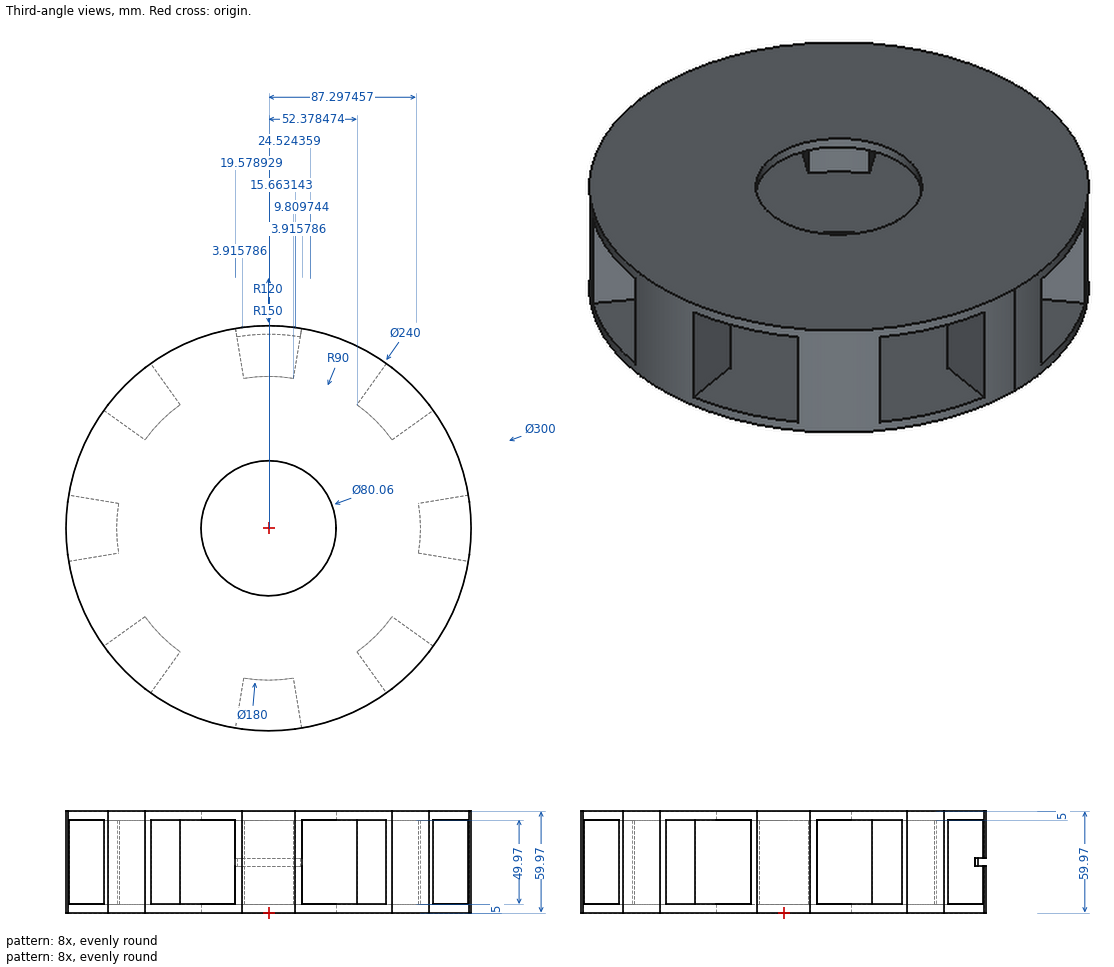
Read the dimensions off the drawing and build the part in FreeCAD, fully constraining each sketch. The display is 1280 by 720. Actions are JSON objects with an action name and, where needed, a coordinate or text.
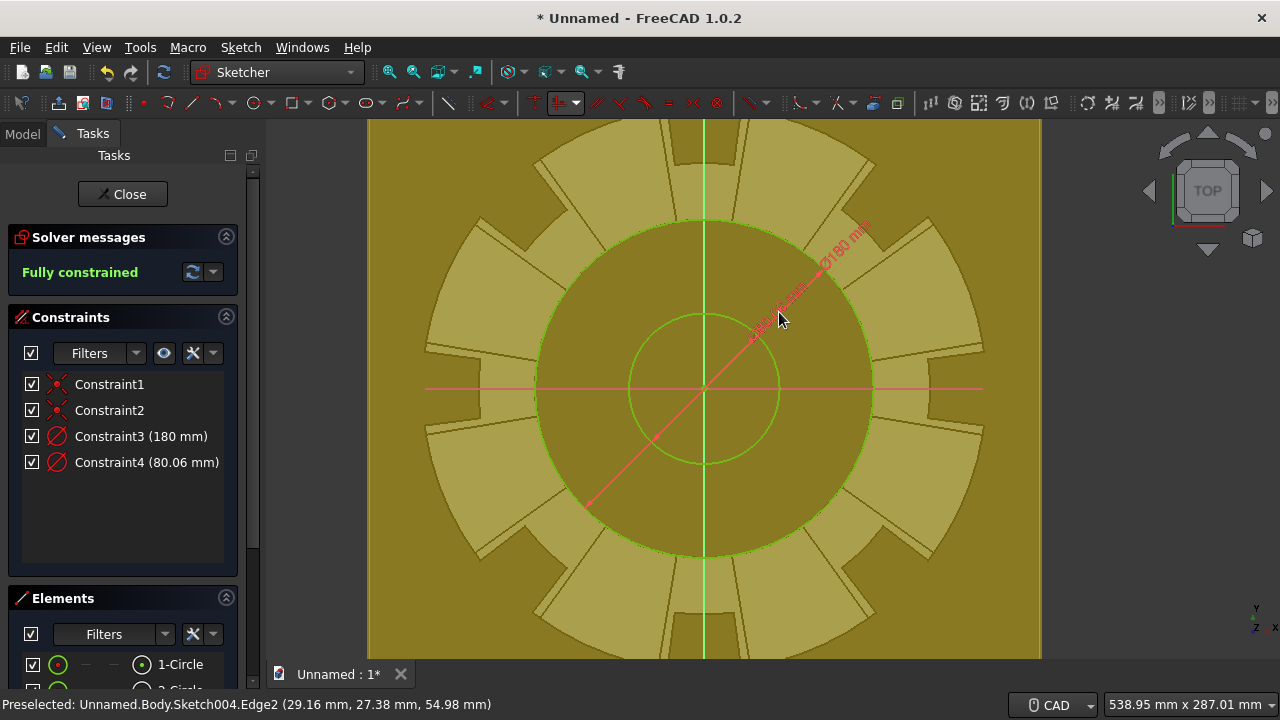
{"action": "left_click", "coordinate": [123, 194]}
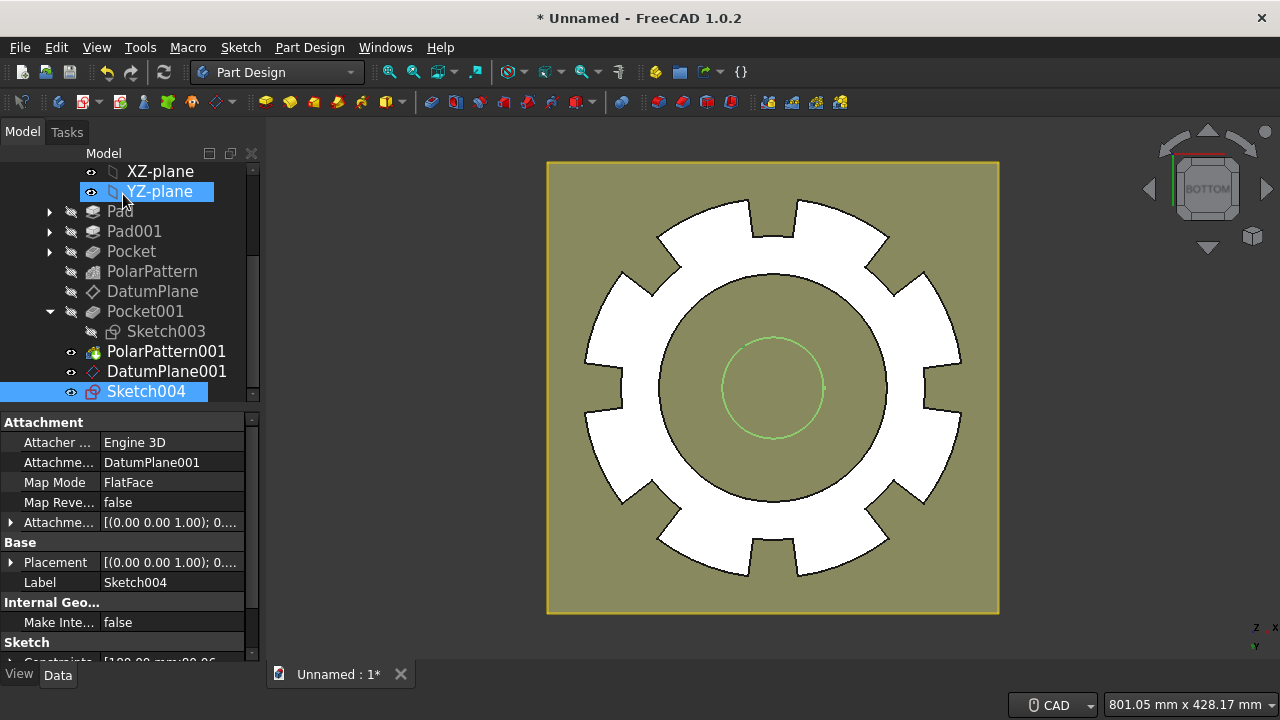
{"action": "left_click", "coordinate": [266, 102]}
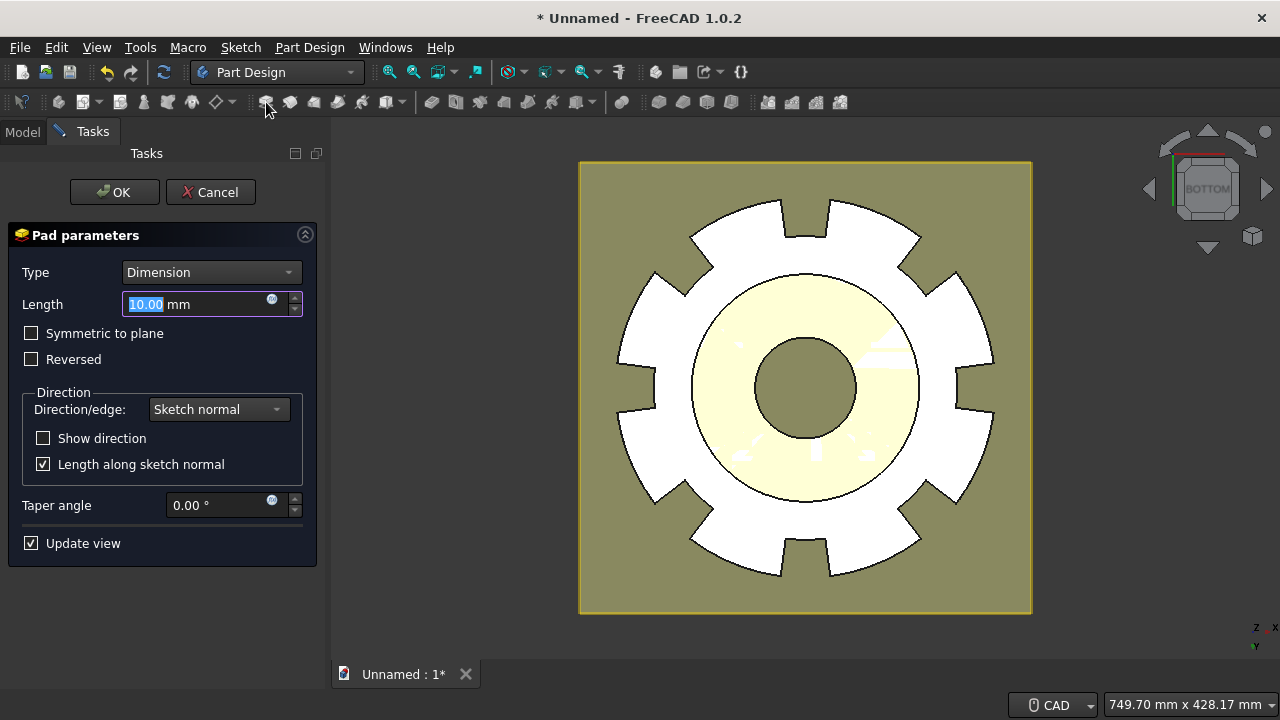
{"action": "type", "text": "5"}
{"action": "key", "text": "Tab"}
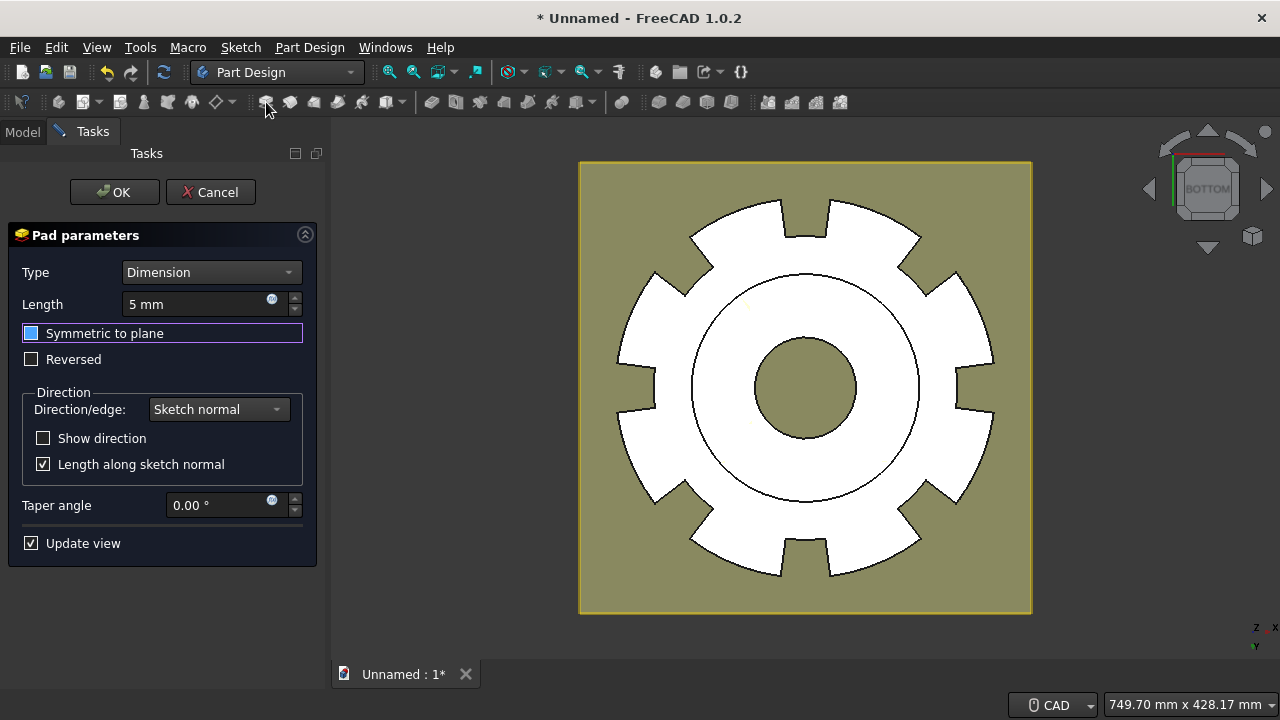
{"action": "left_click", "coordinate": [115, 192]}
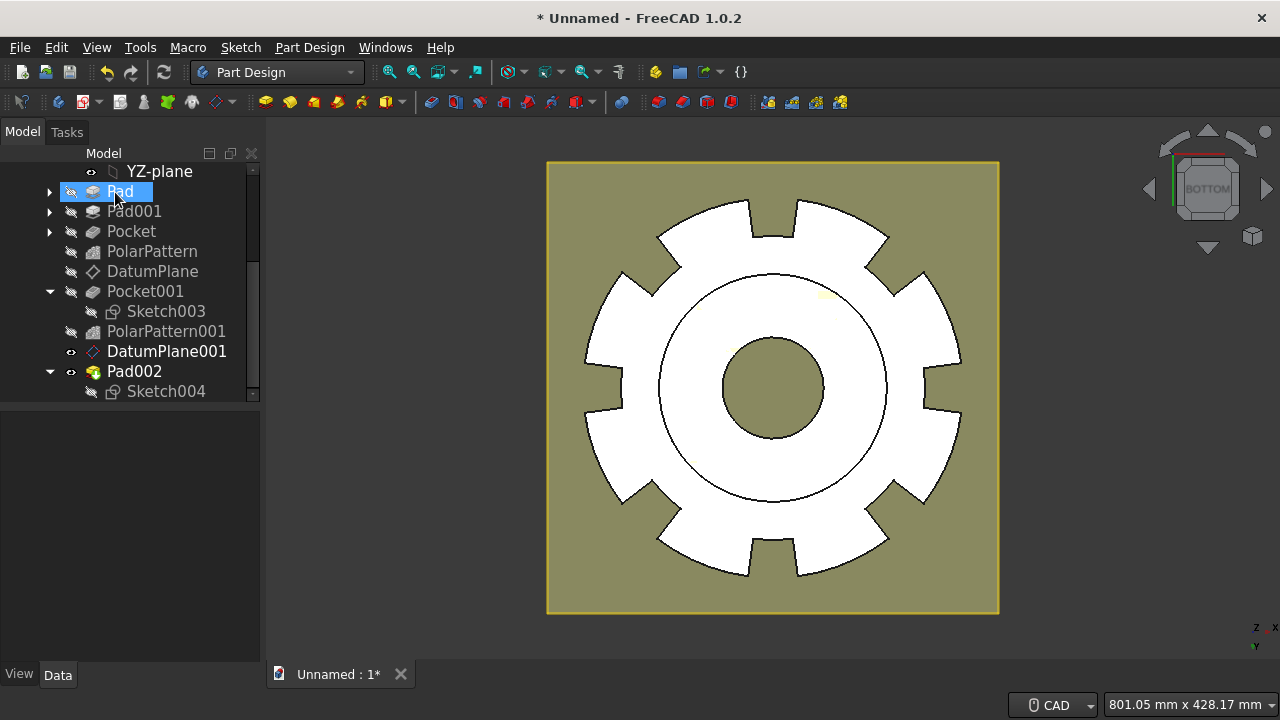
{"action": "left_click", "coordinate": [116, 352]}
{"action": "key", "text": "space"}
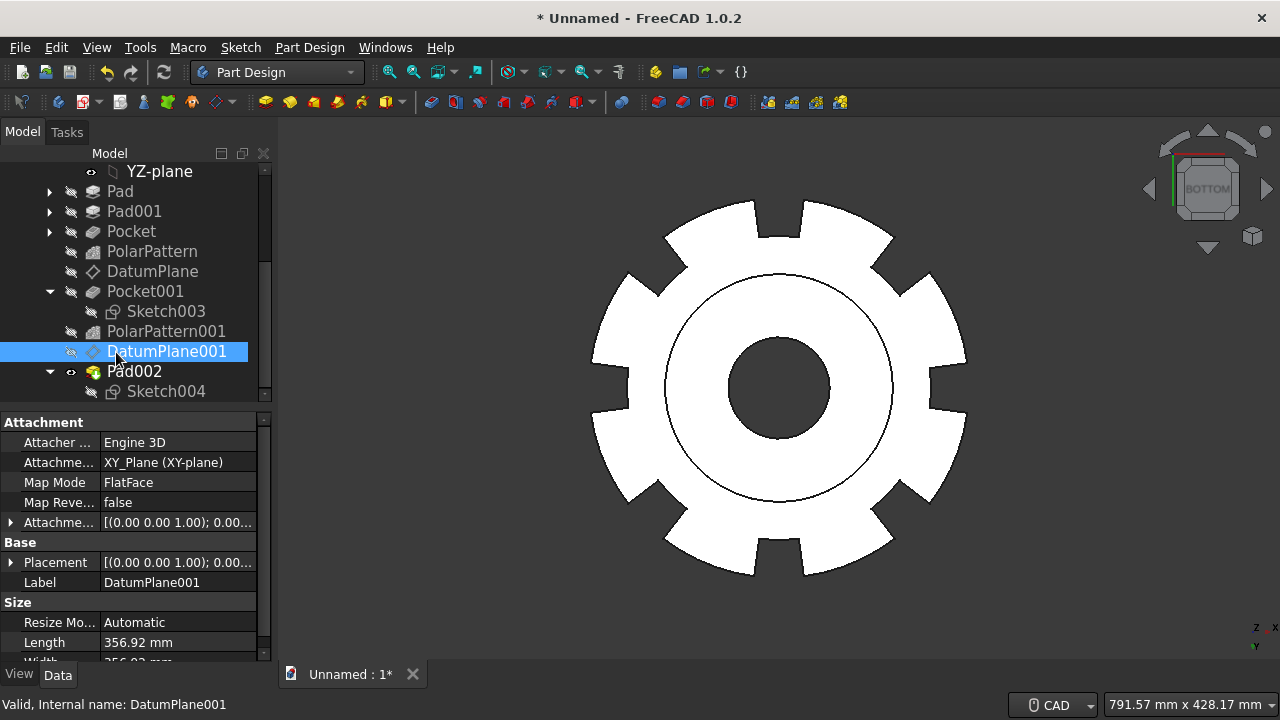
{"action": "left_click", "coordinate": [318, 619]}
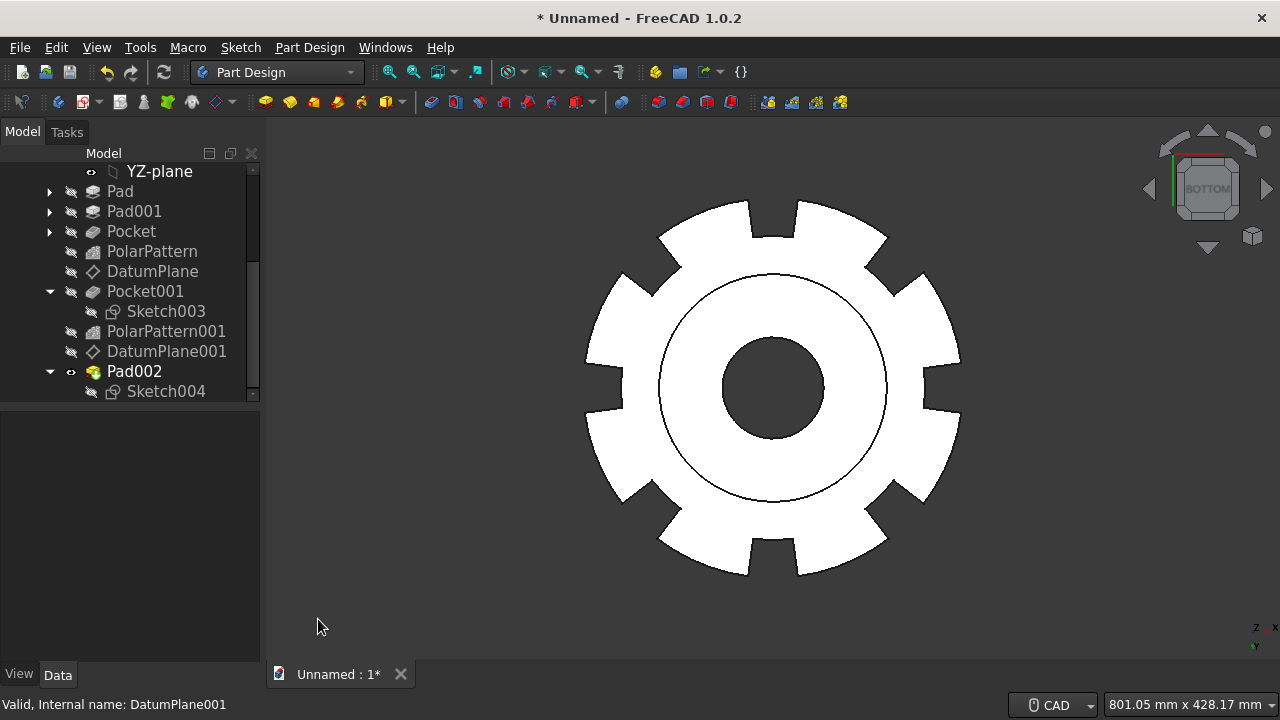
{"action": "left_click", "coordinate": [84, 102]}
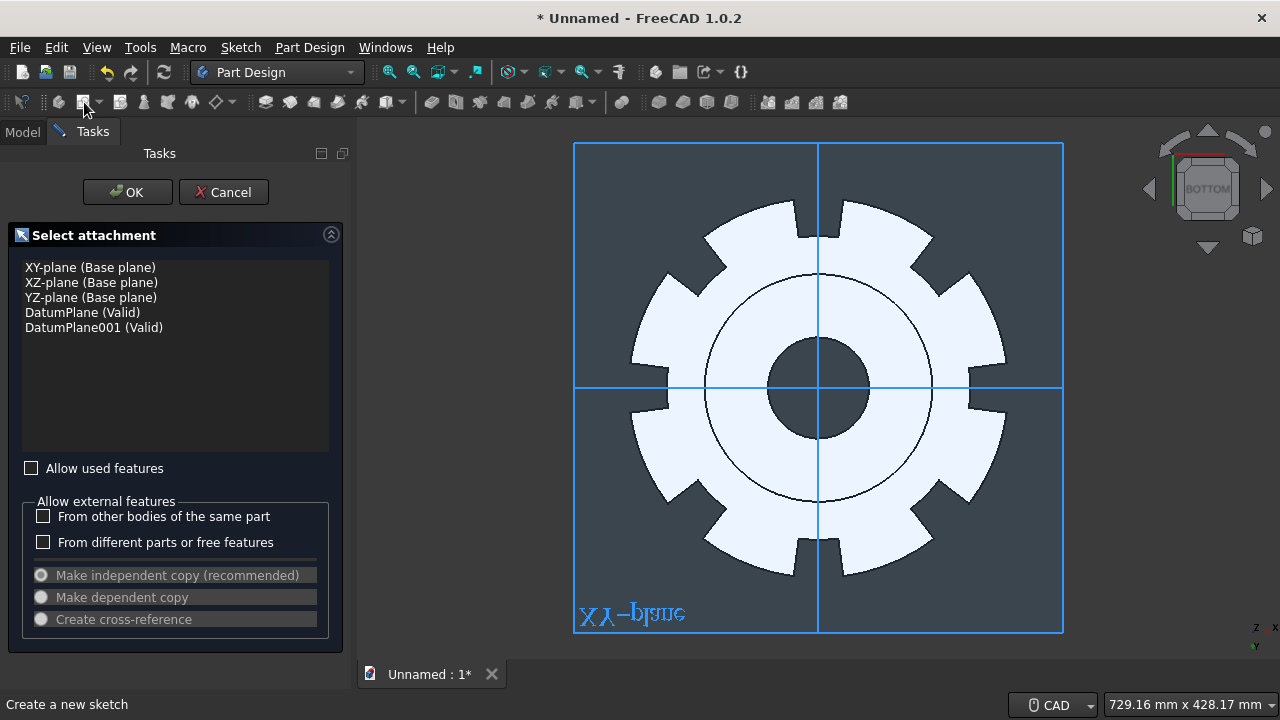
{"action": "left_click", "coordinate": [82, 268]}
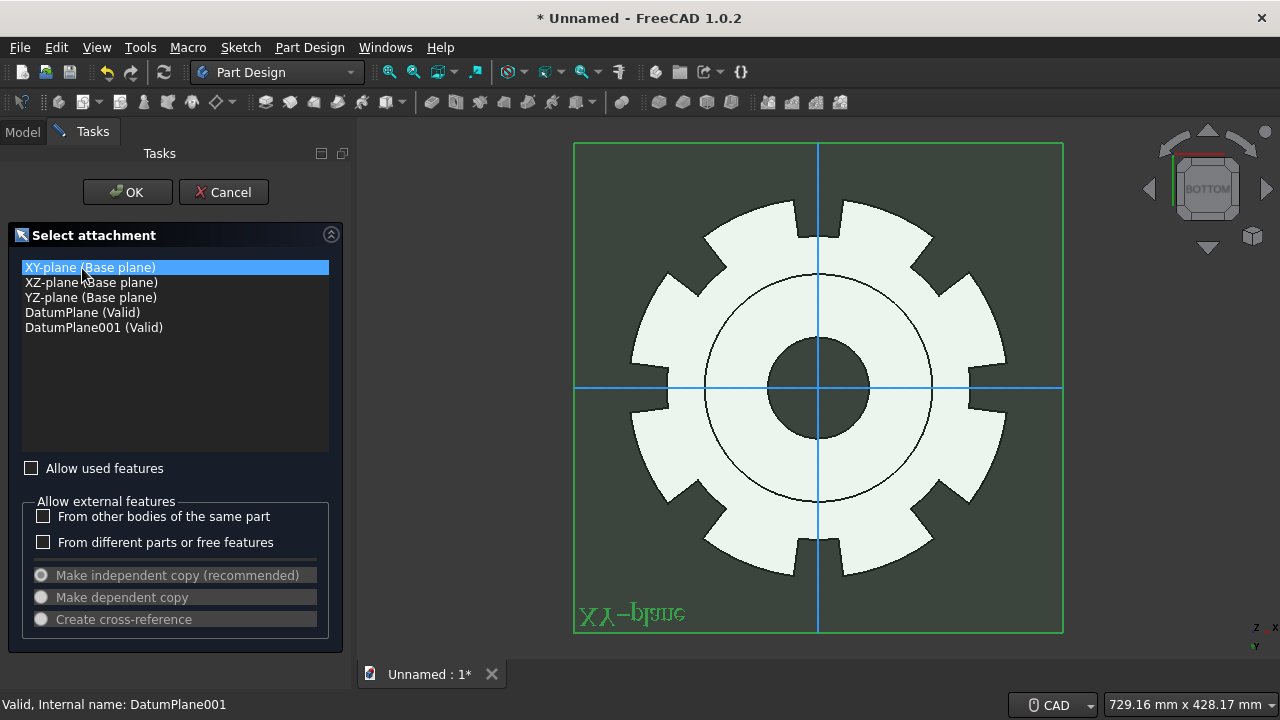
{"action": "left_click", "coordinate": [128, 192]}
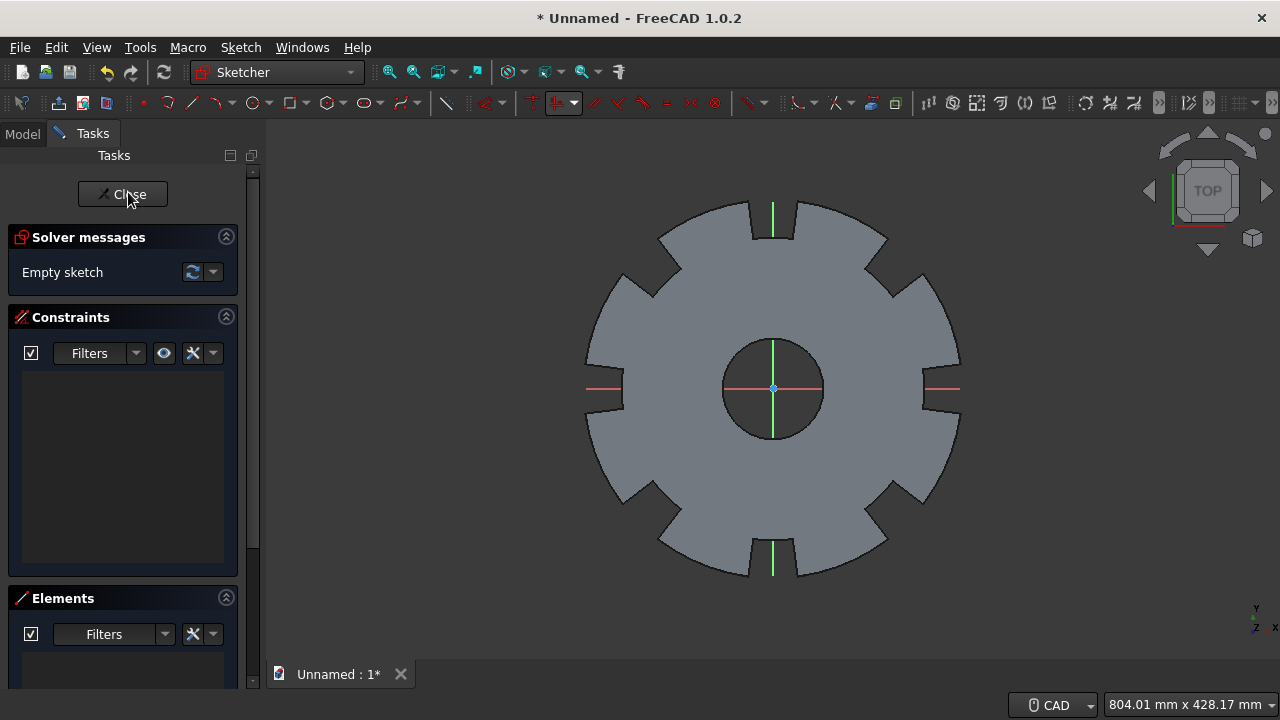
{"action": "key", "text": "q s"}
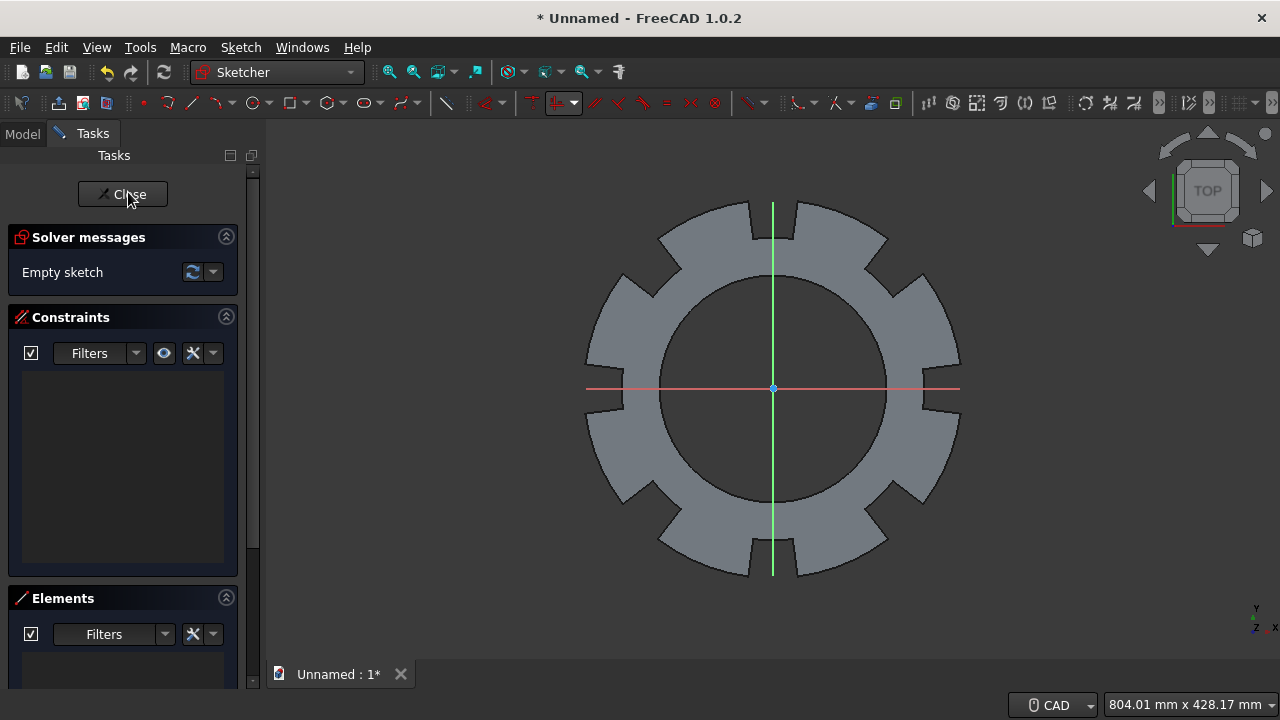
{"action": "scroll", "coordinate": [912, 389], "scroll_direction": "up", "scroll_amount": 2}